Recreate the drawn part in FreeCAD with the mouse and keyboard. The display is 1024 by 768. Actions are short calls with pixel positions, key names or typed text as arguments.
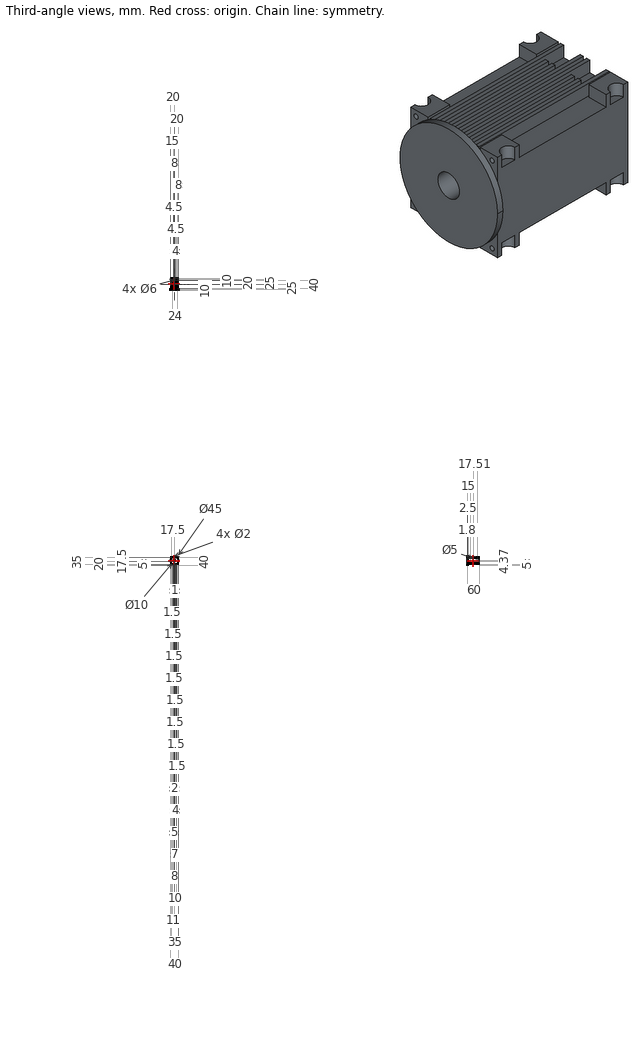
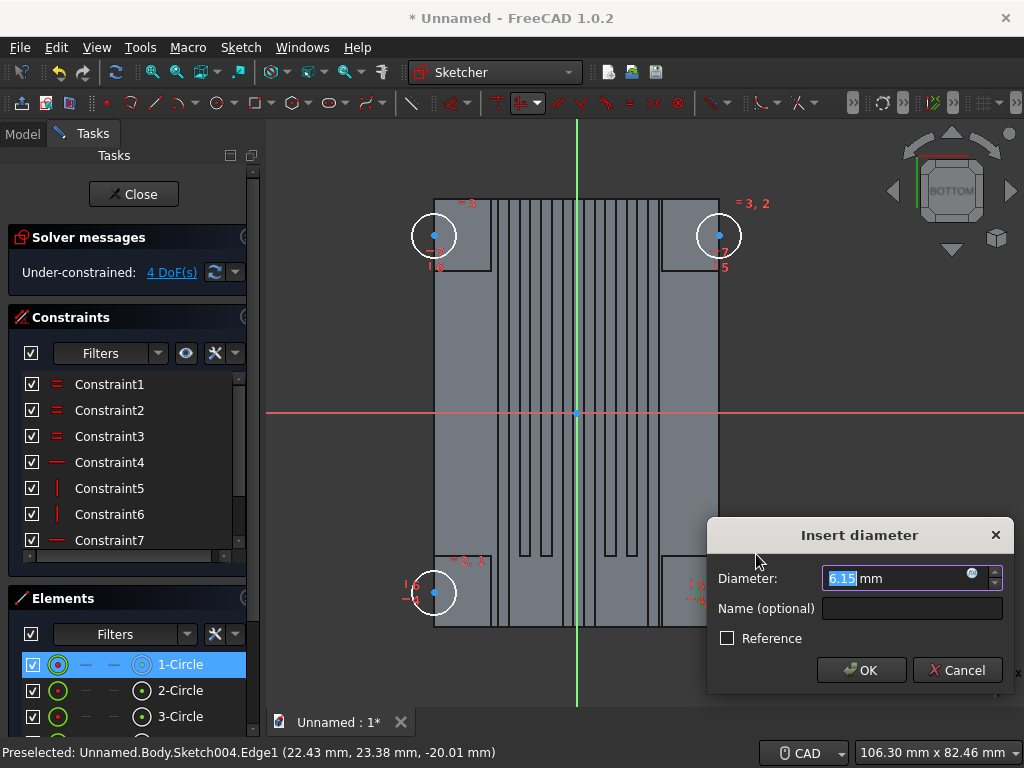
text(6)
key(Return)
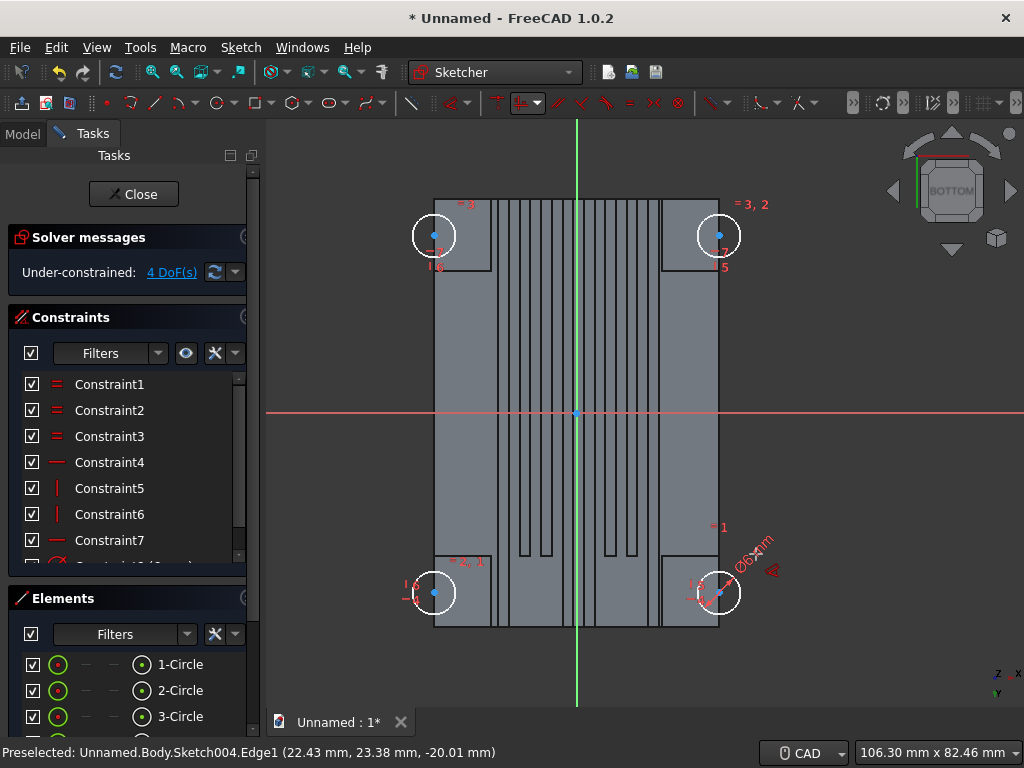
click(719, 593)
click(648, 627)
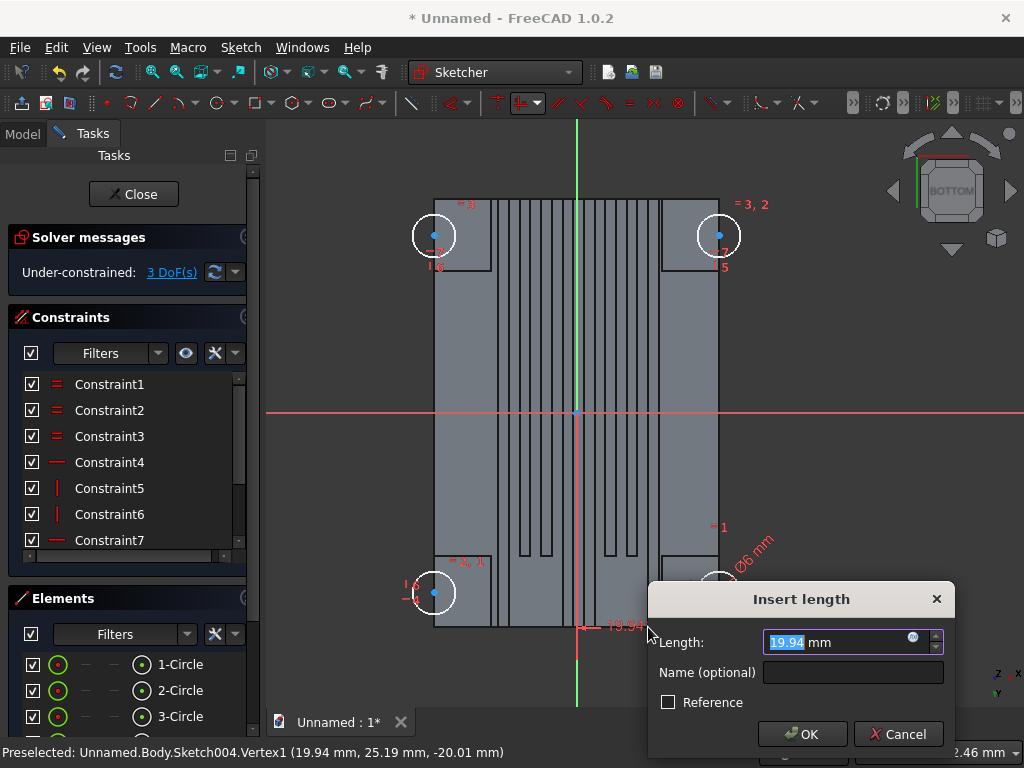
text(20)
key(Return)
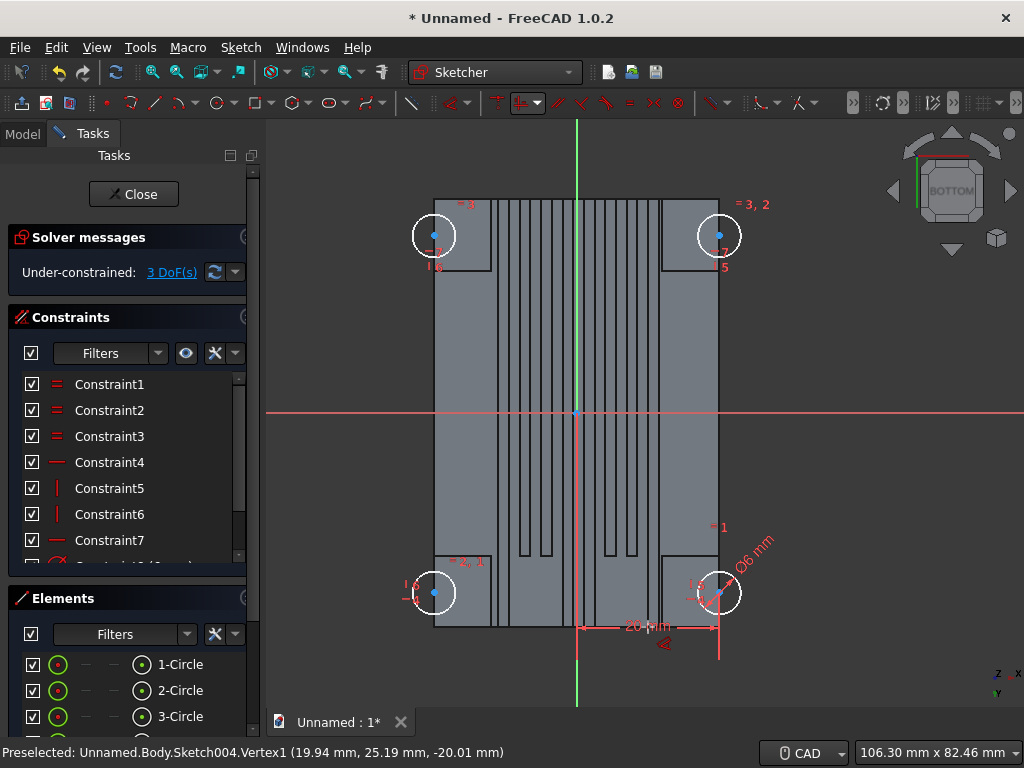
click(719, 593)
click(753, 503)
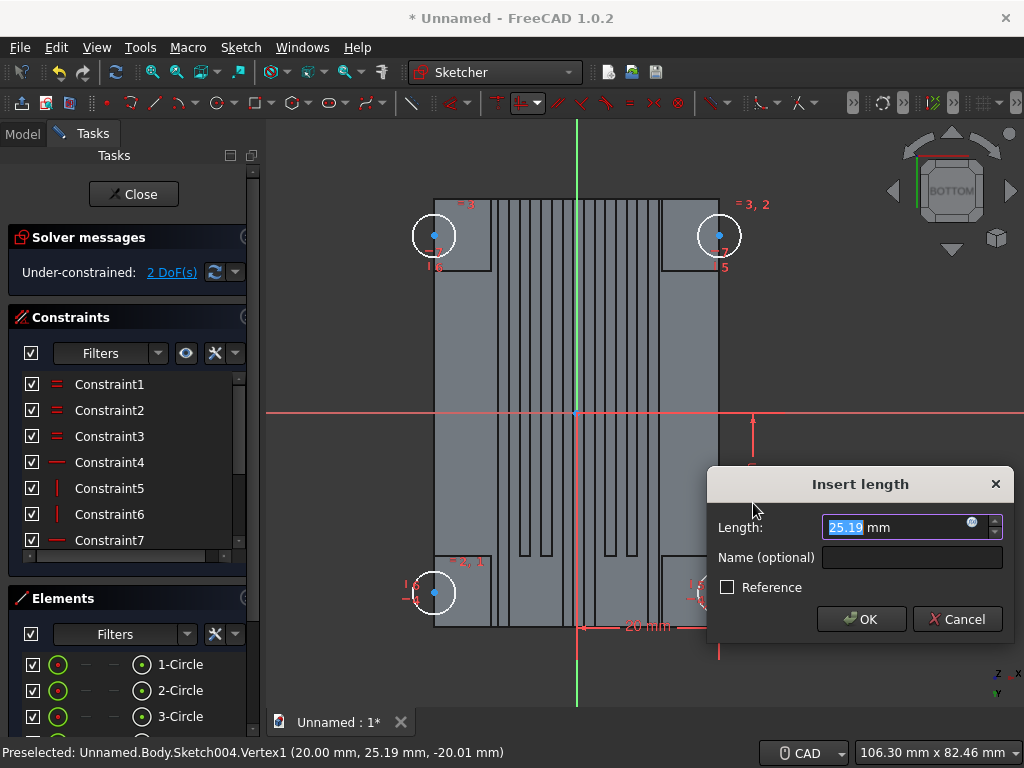
text(25)
key(Return)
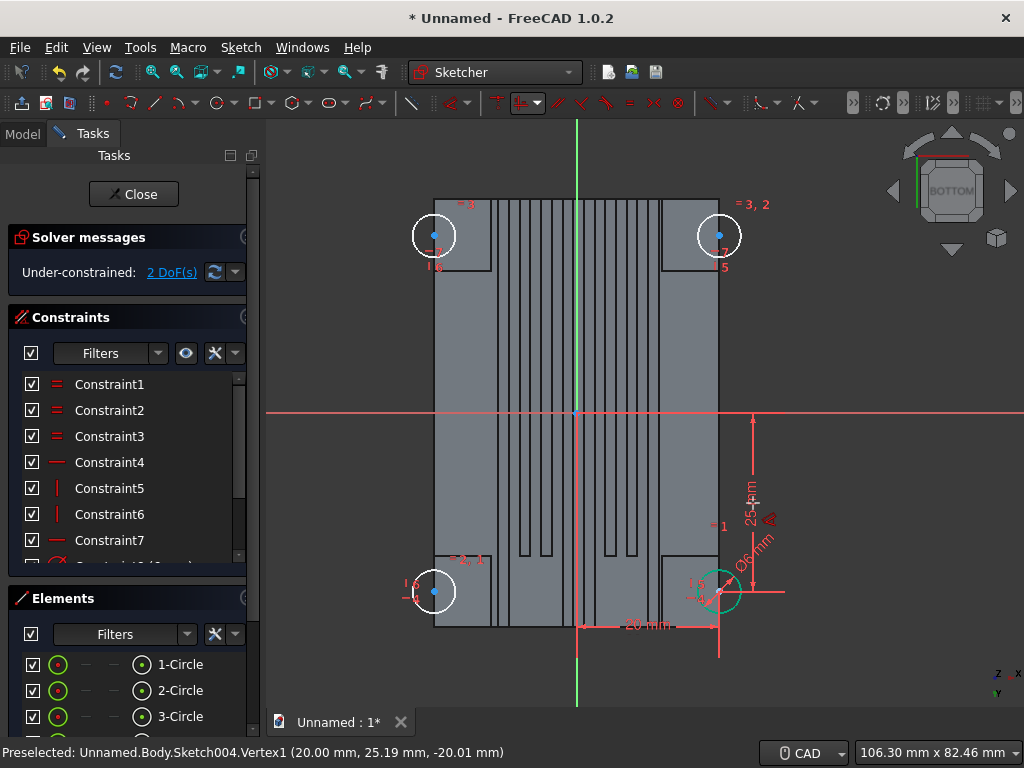
click(434, 592)
click(505, 626)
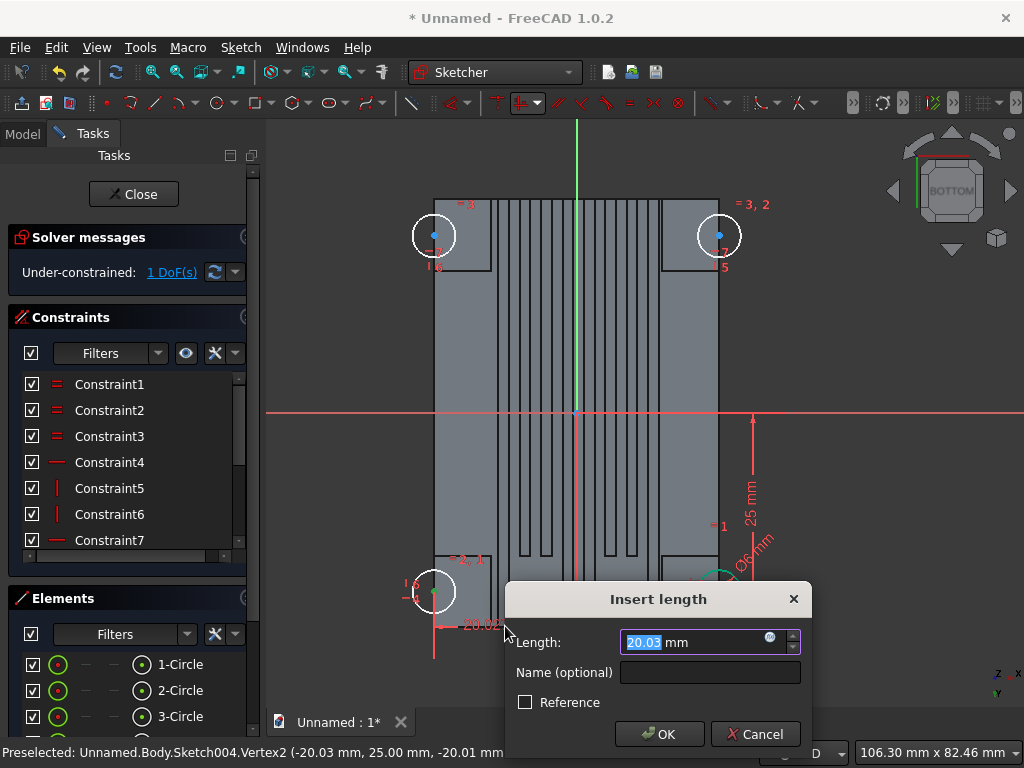
text(20)
key(Return)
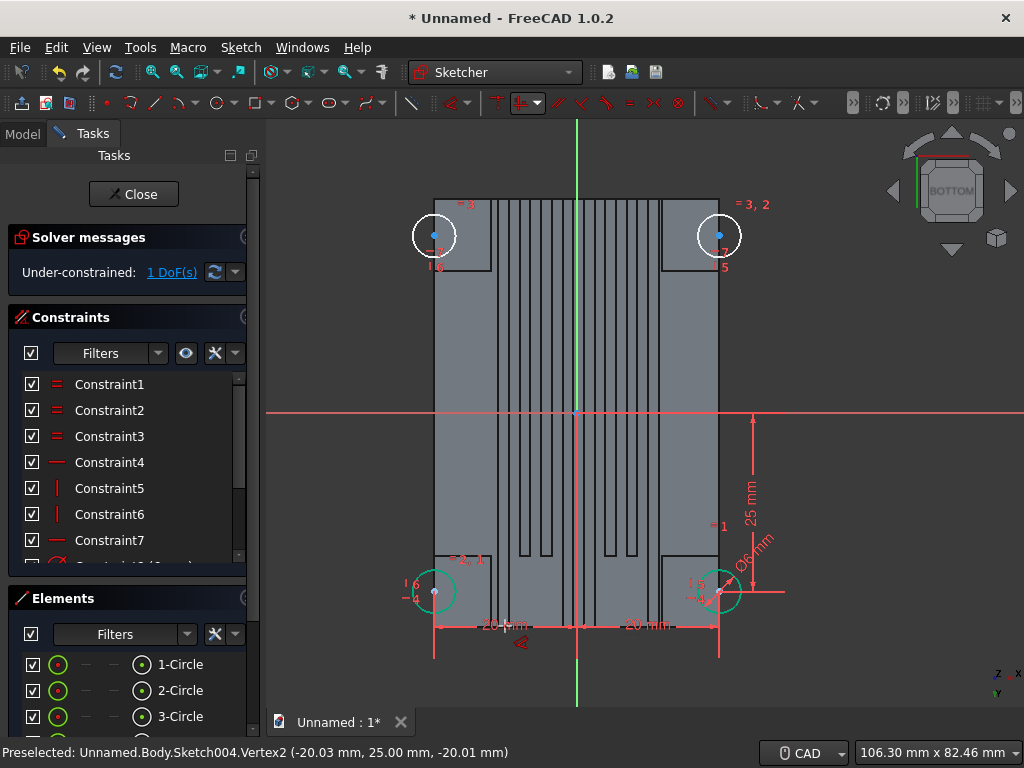
click(719, 236)
click(753, 325)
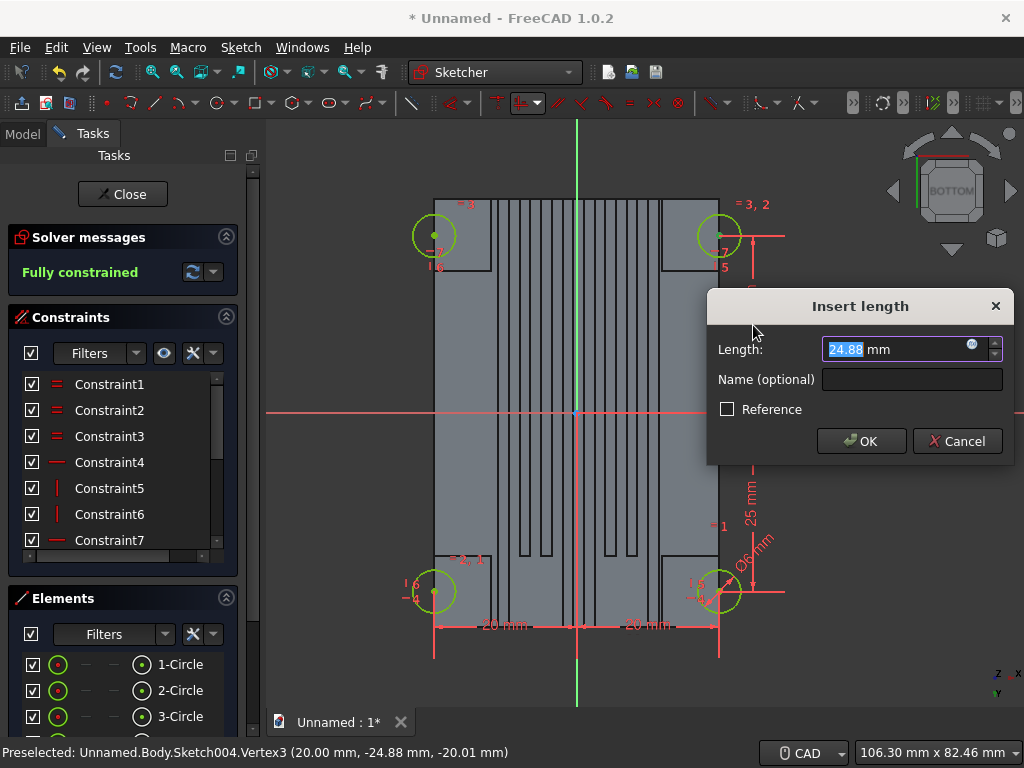
text(25)
key(Return)
key(Escape)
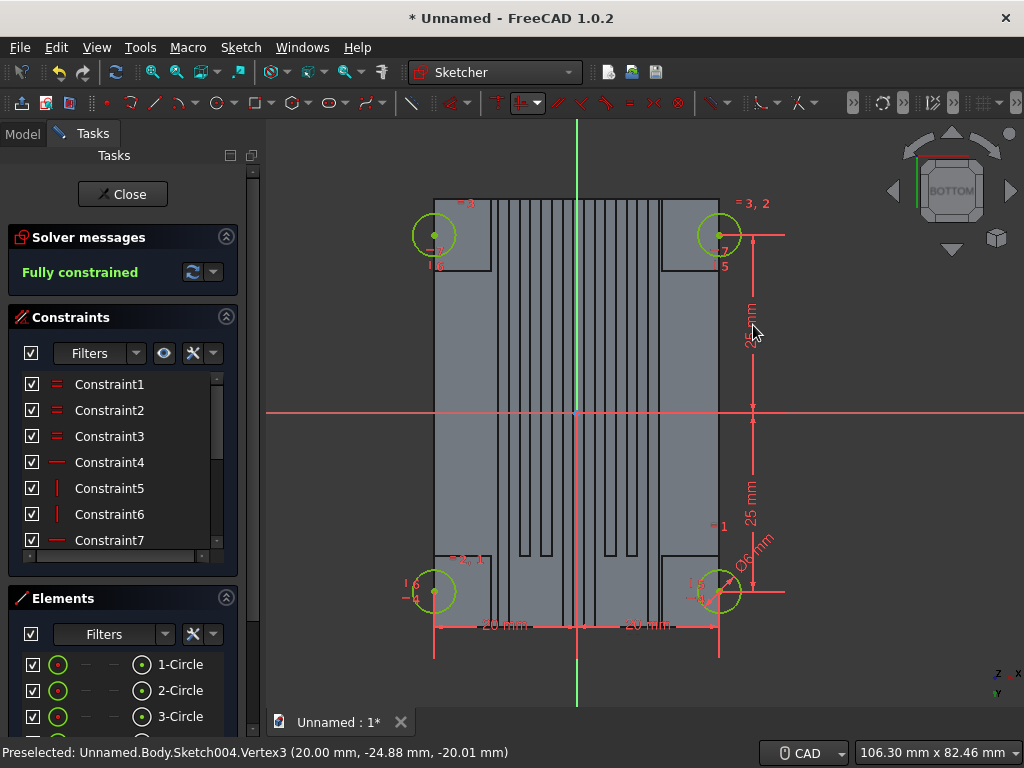
click(123, 194)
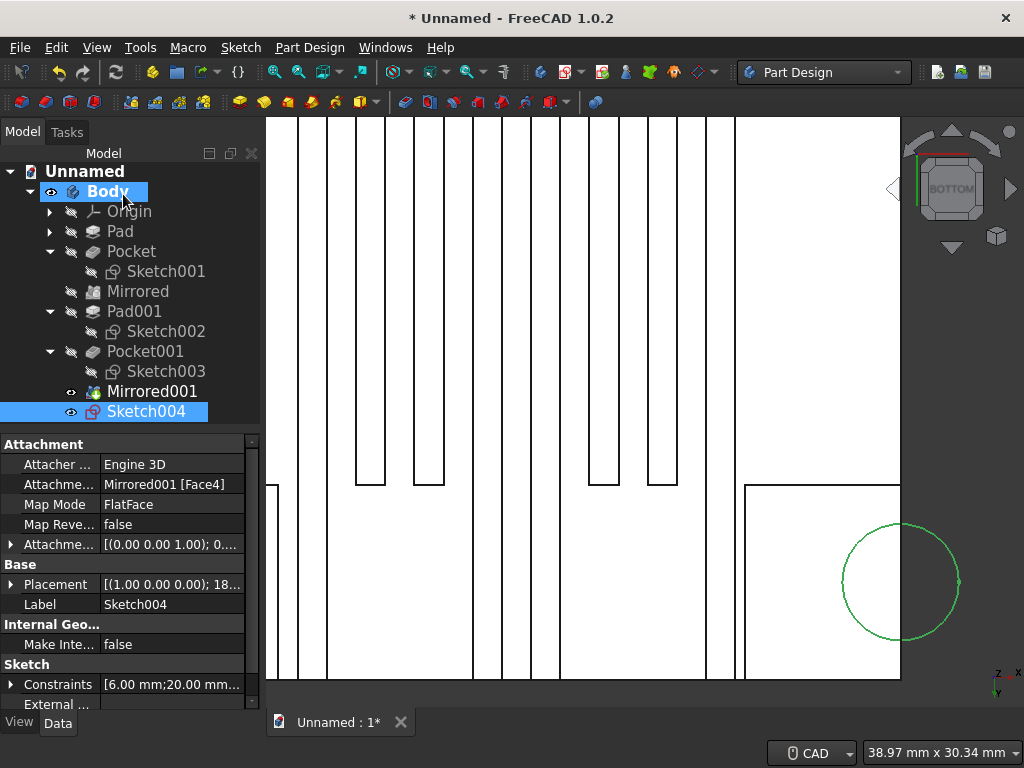
click(406, 102)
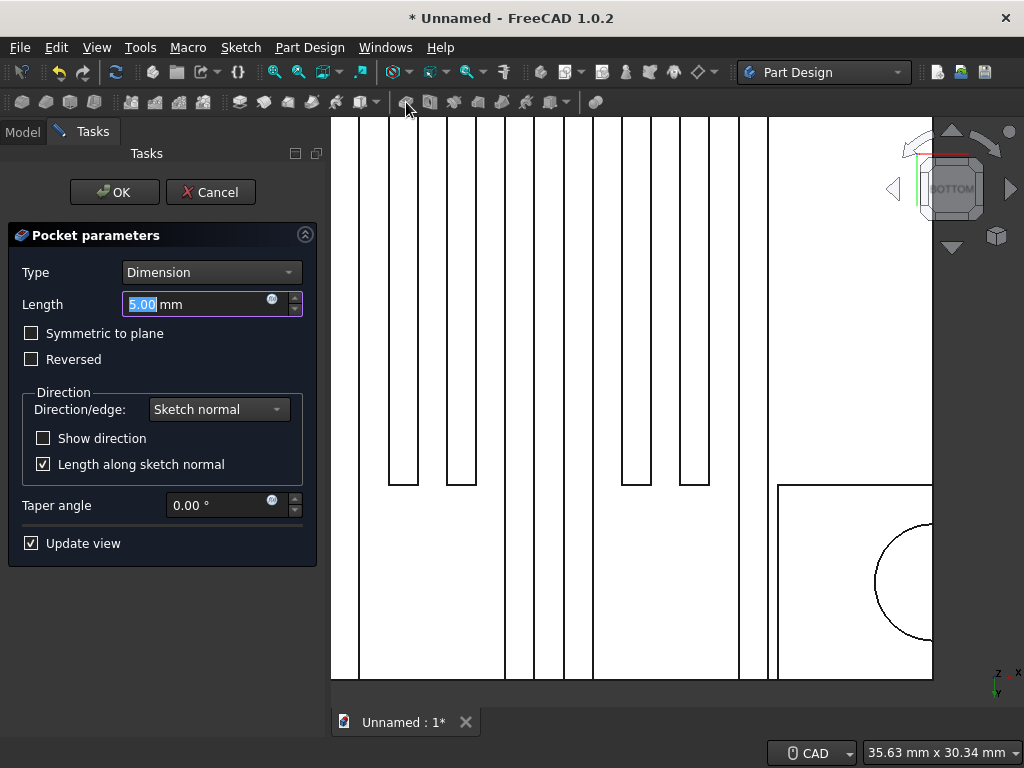
text(5)
key(Tab)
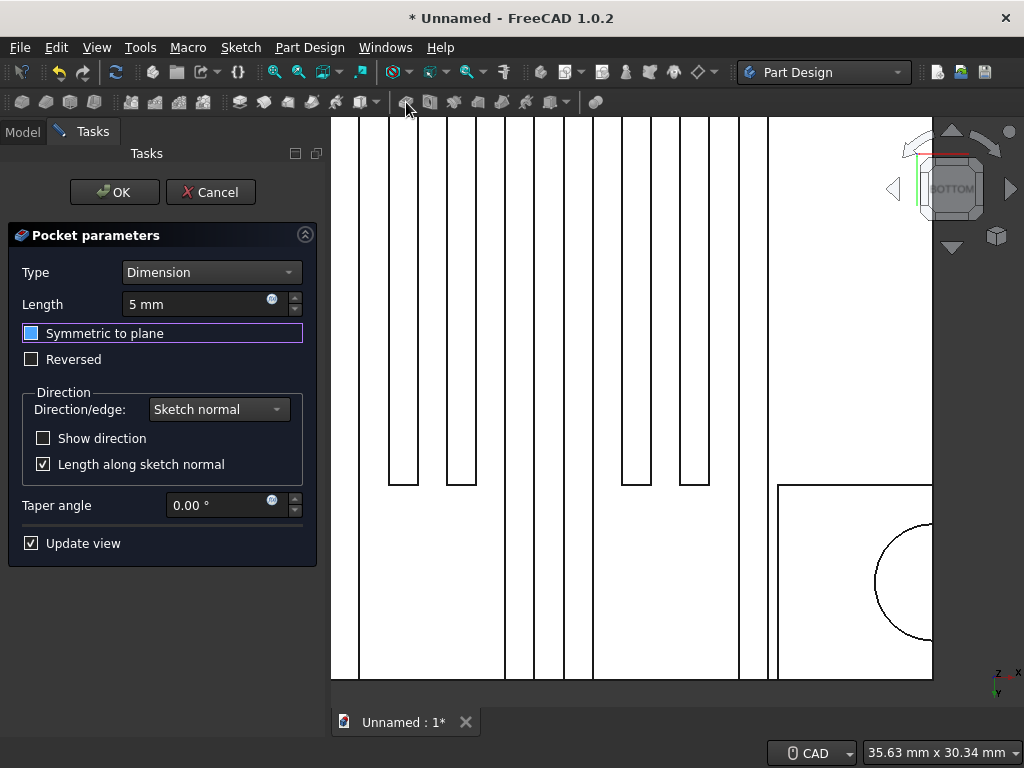
click(115, 192)